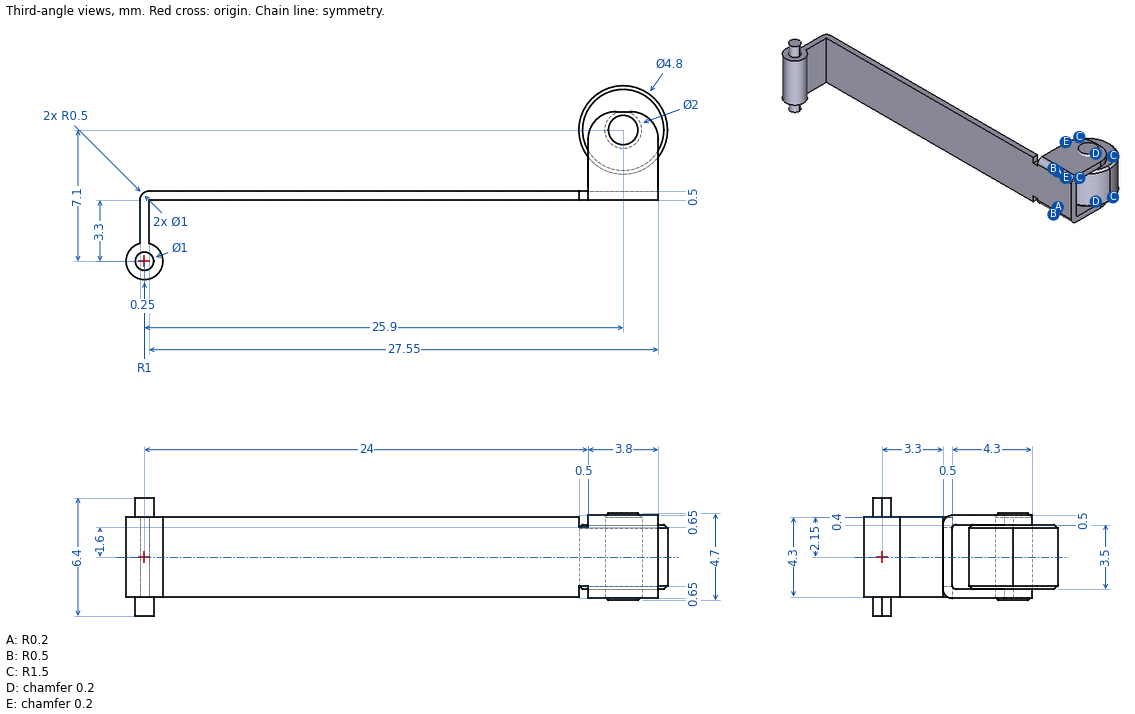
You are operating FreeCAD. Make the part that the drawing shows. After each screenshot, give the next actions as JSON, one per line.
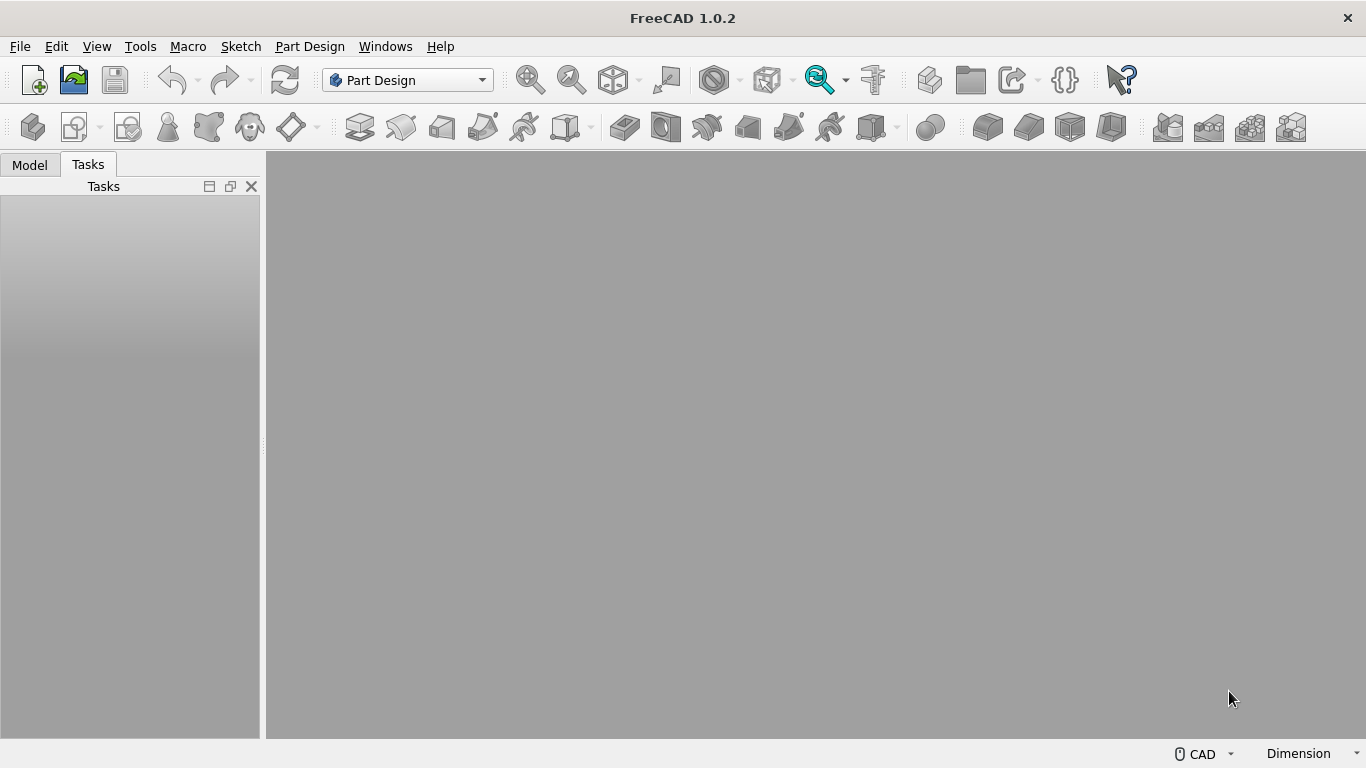
{"action": "key", "text": "ctrl+n"}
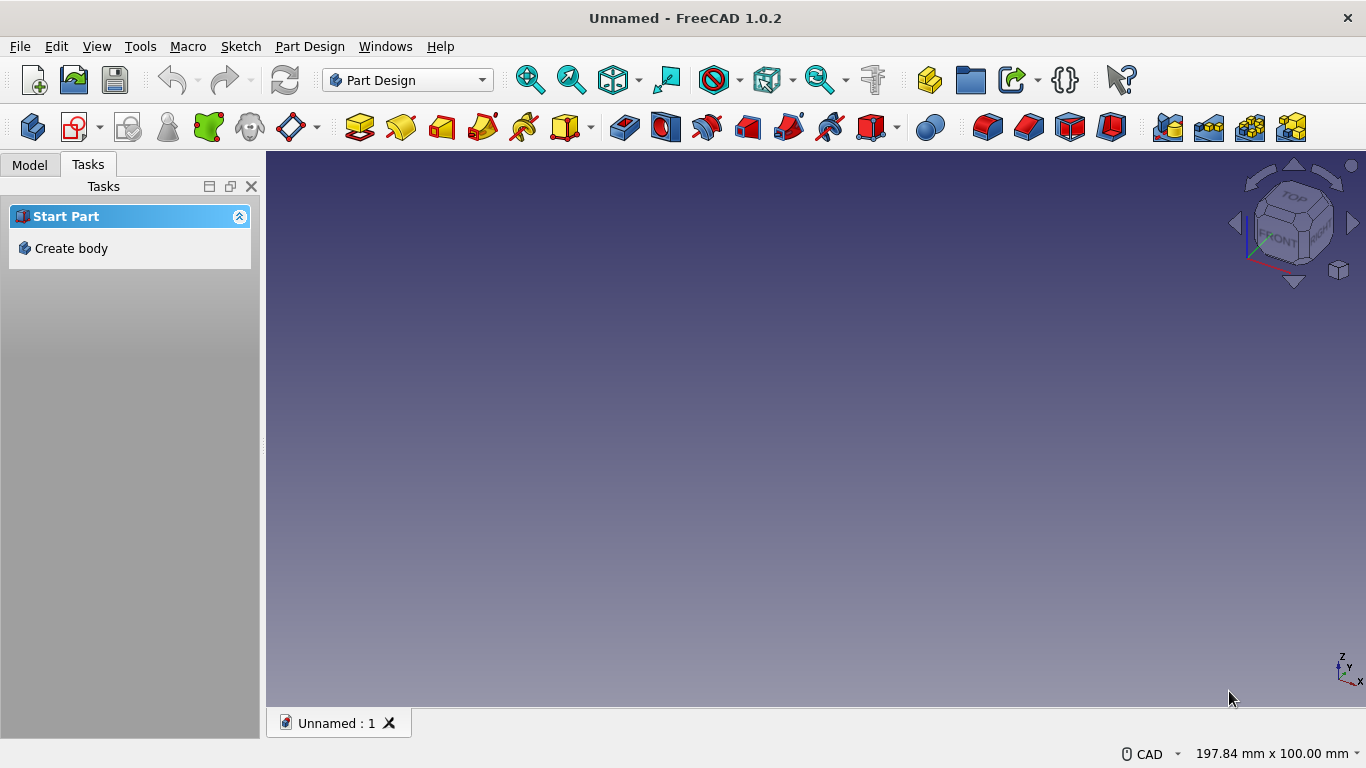
{"action": "left_click", "coordinate": [74, 128]}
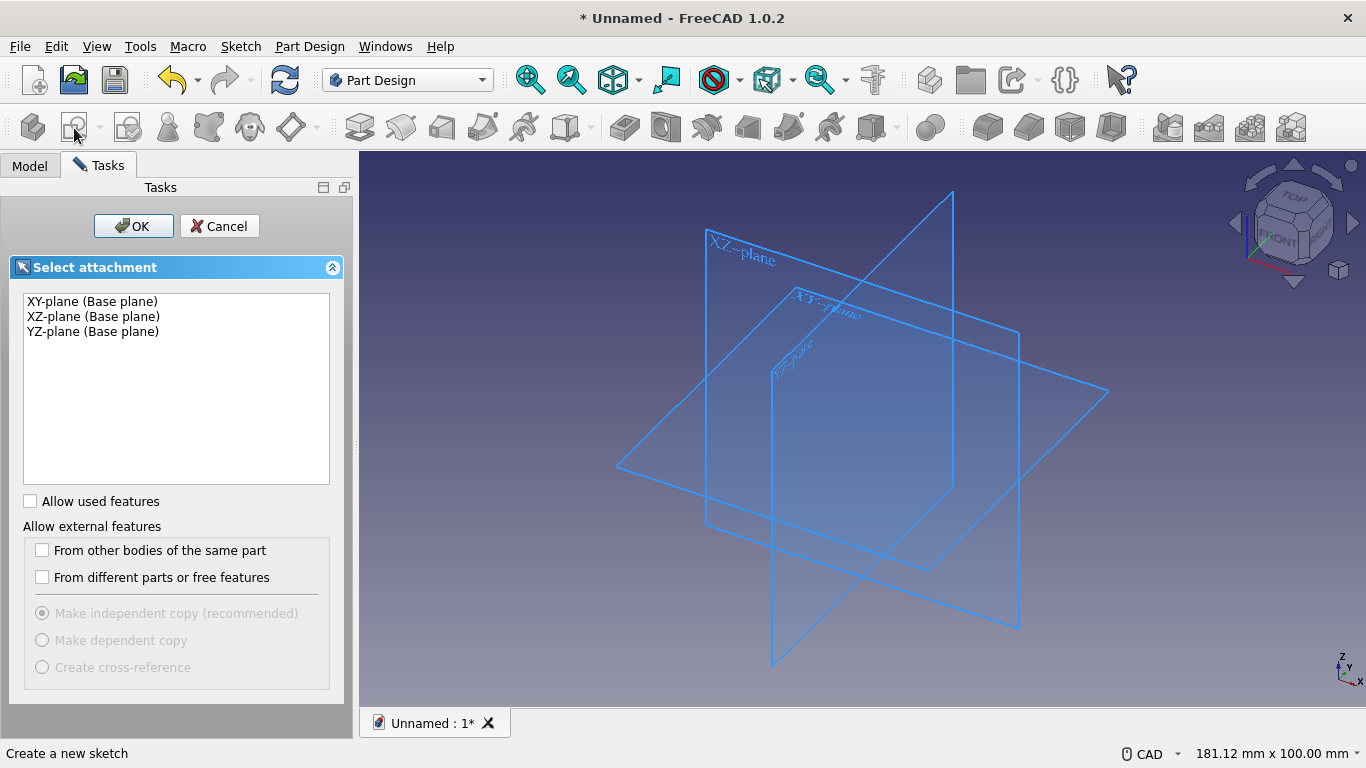
{"action": "left_click", "coordinate": [84, 302]}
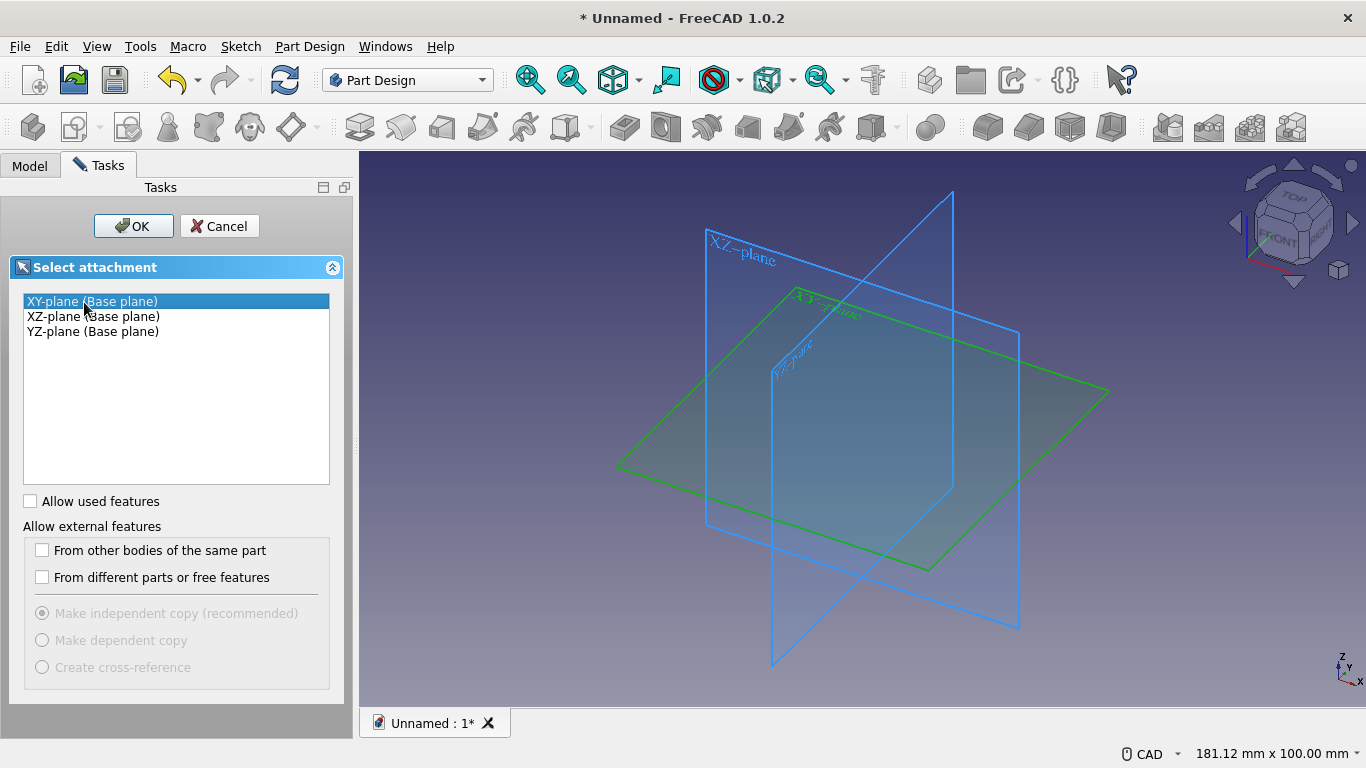
{"action": "left_click", "coordinate": [134, 226]}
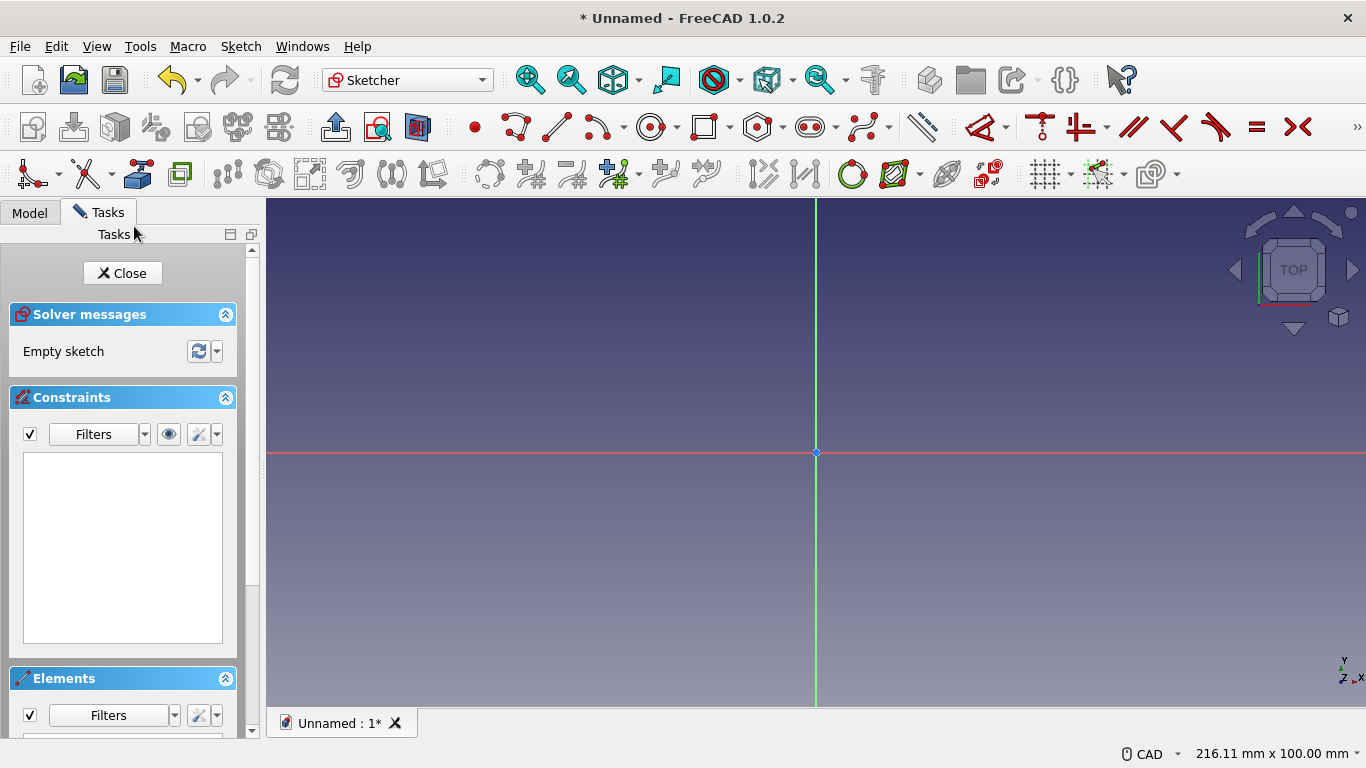
{"action": "scroll", "coordinate": [931, 443], "scroll_direction": "up", "scroll_amount": 7}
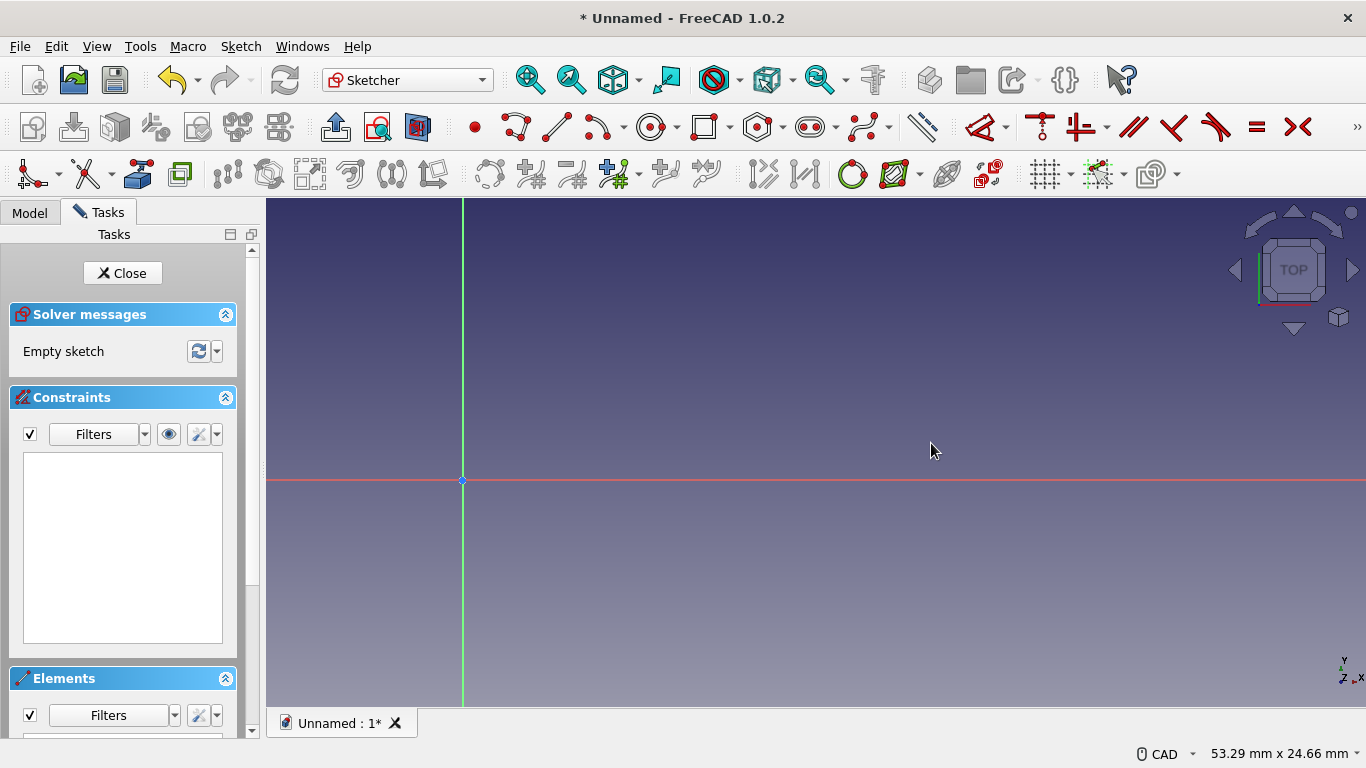
{"action": "key", "text": "g l"}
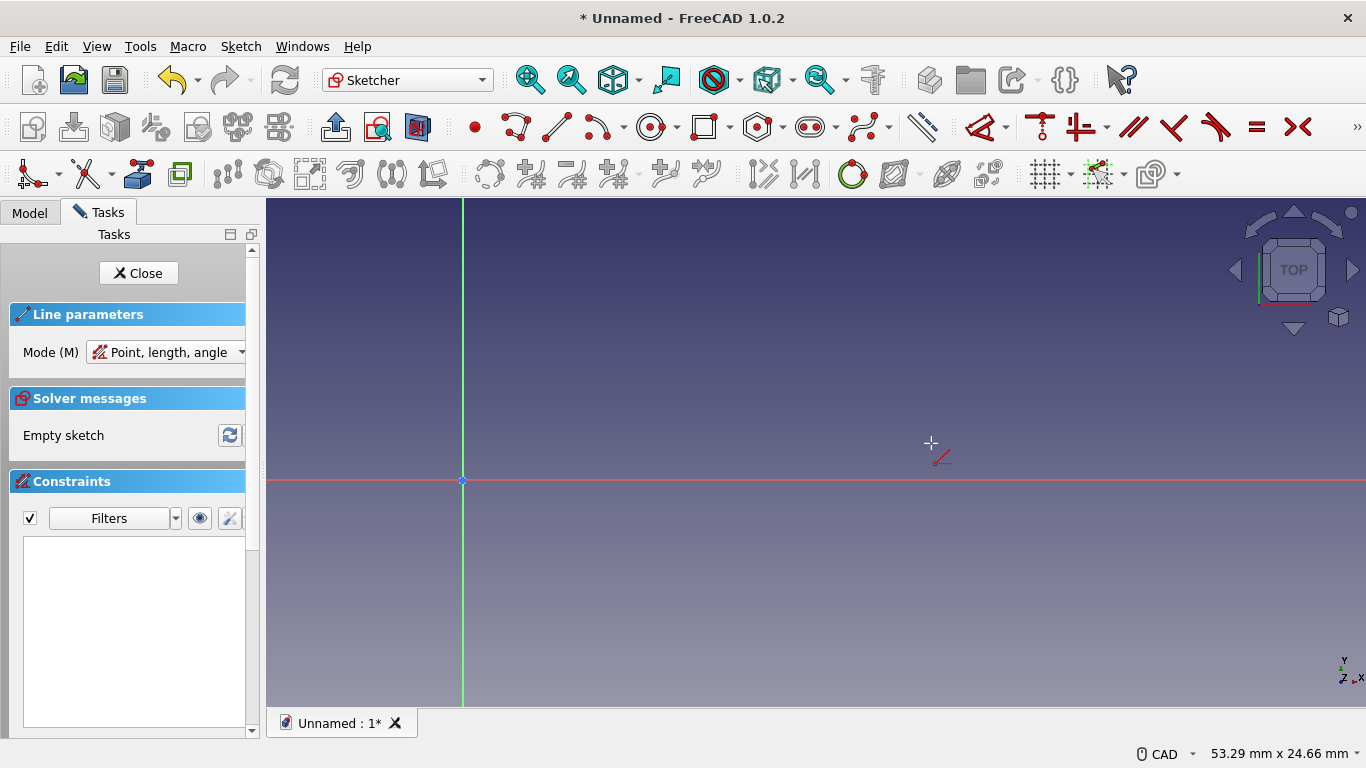
{"action": "scroll", "coordinate": [458, 412], "scroll_direction": "up", "scroll_amount": 6}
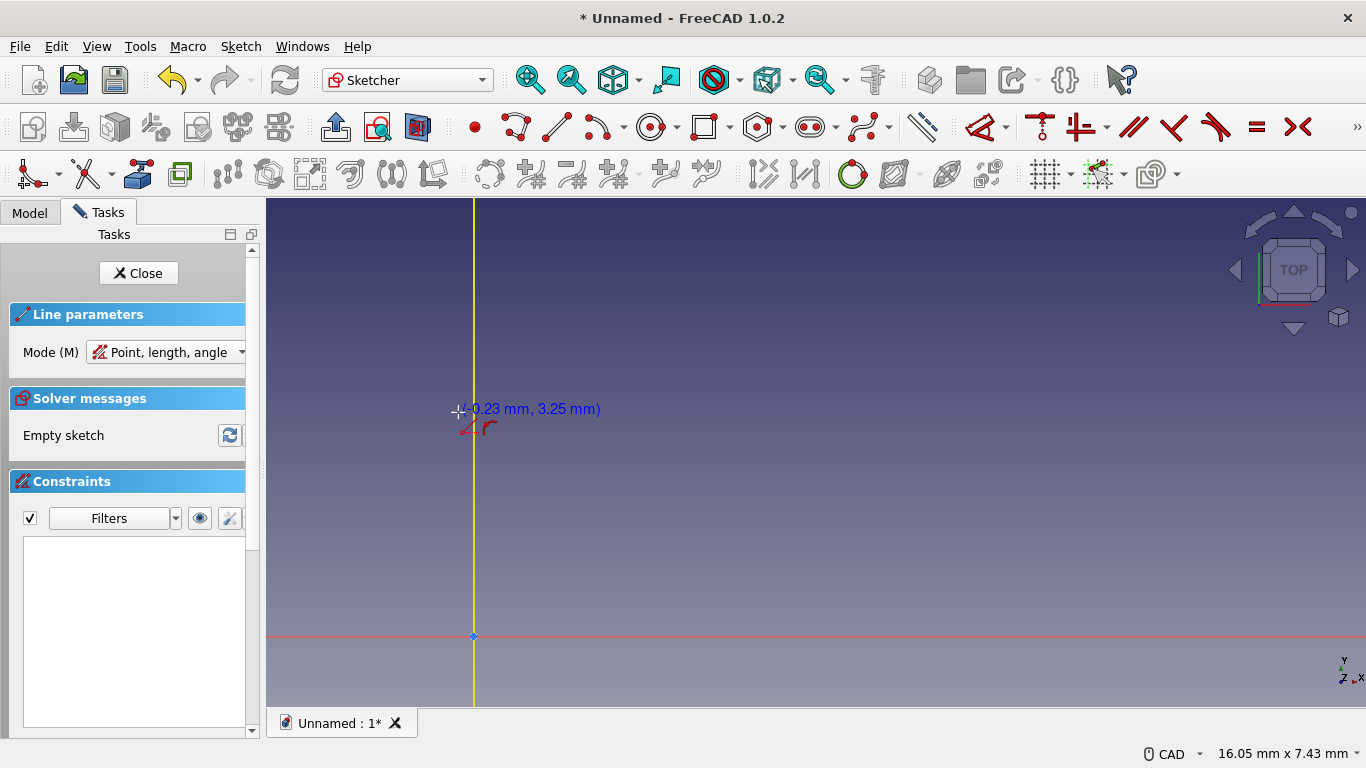
{"action": "left_click", "coordinate": [456, 411]}
{"action": "left_click", "coordinate": [456, 571]}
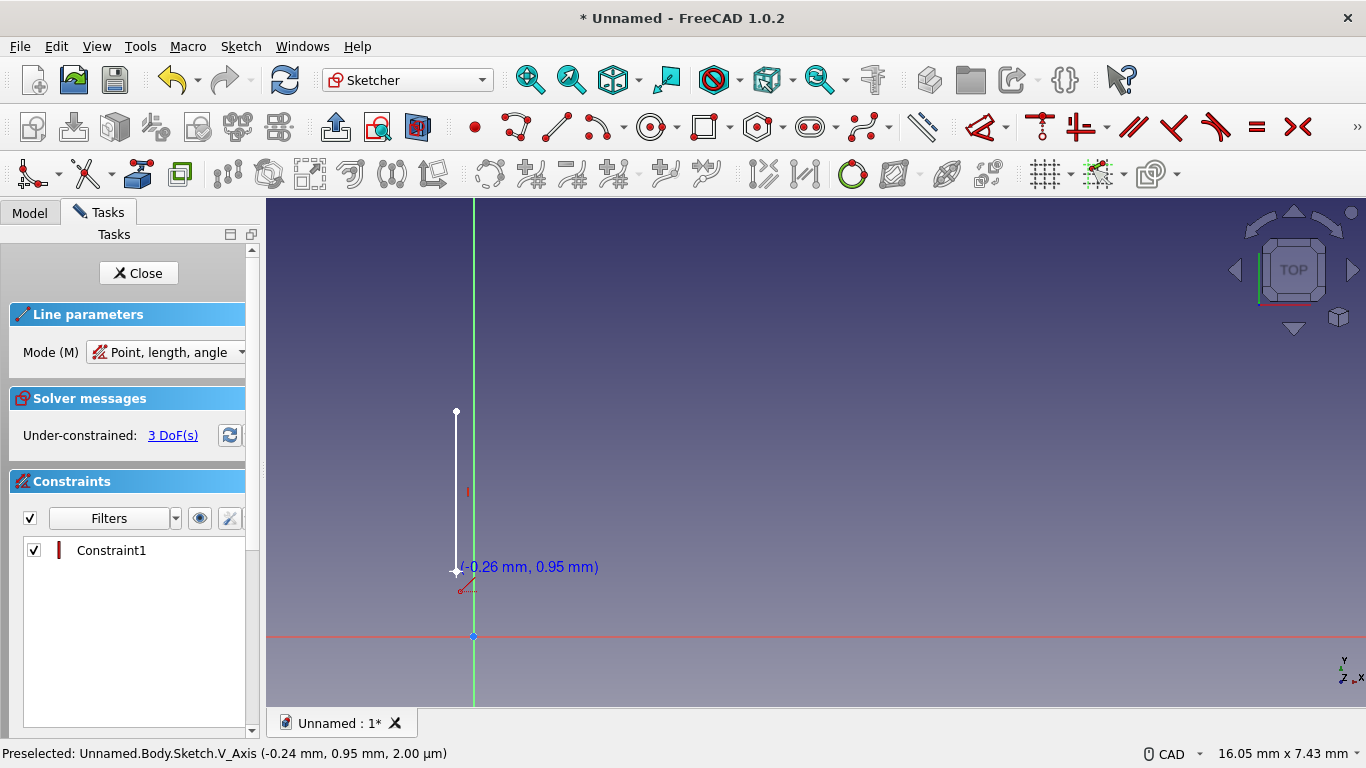
{"action": "left_click", "coordinate": [516, 128]}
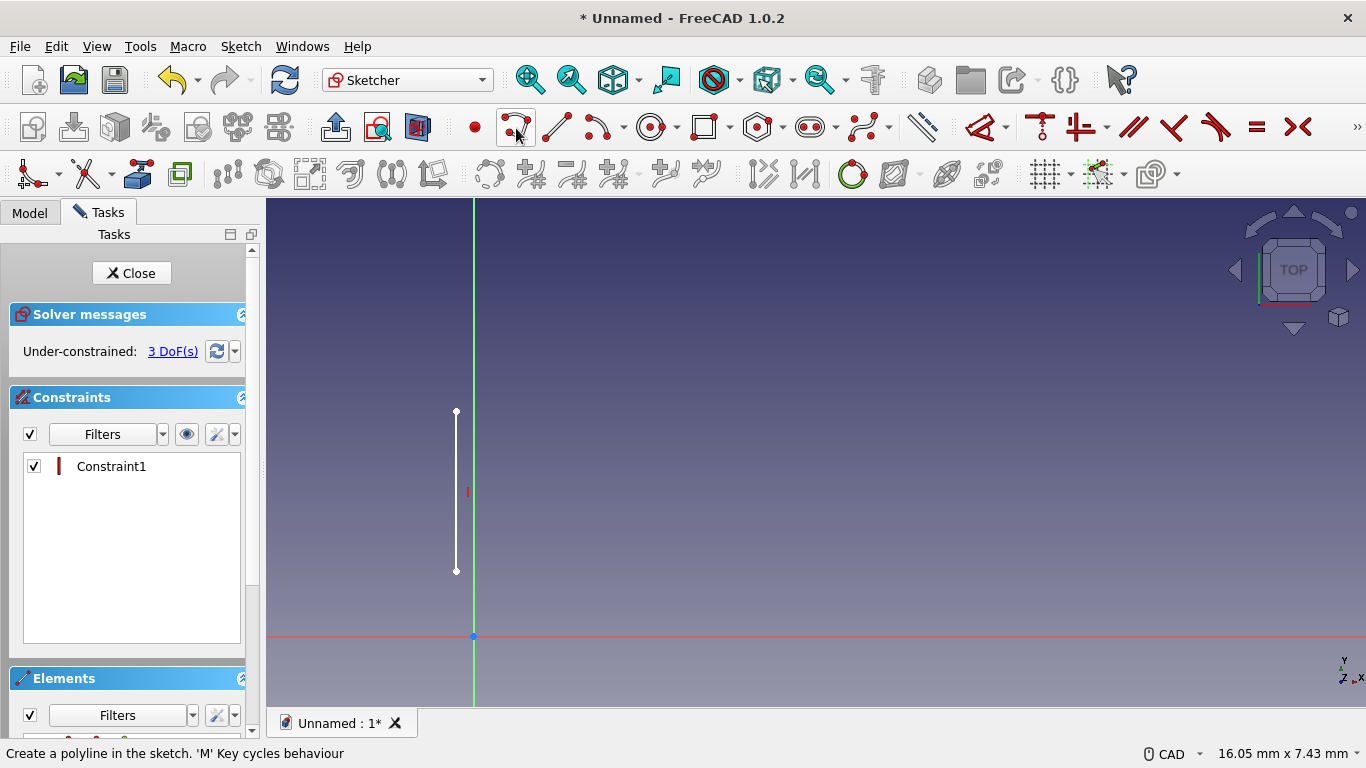
{"action": "left_click", "coordinate": [491, 571]}
{"action": "left_click", "coordinate": [491, 411]}